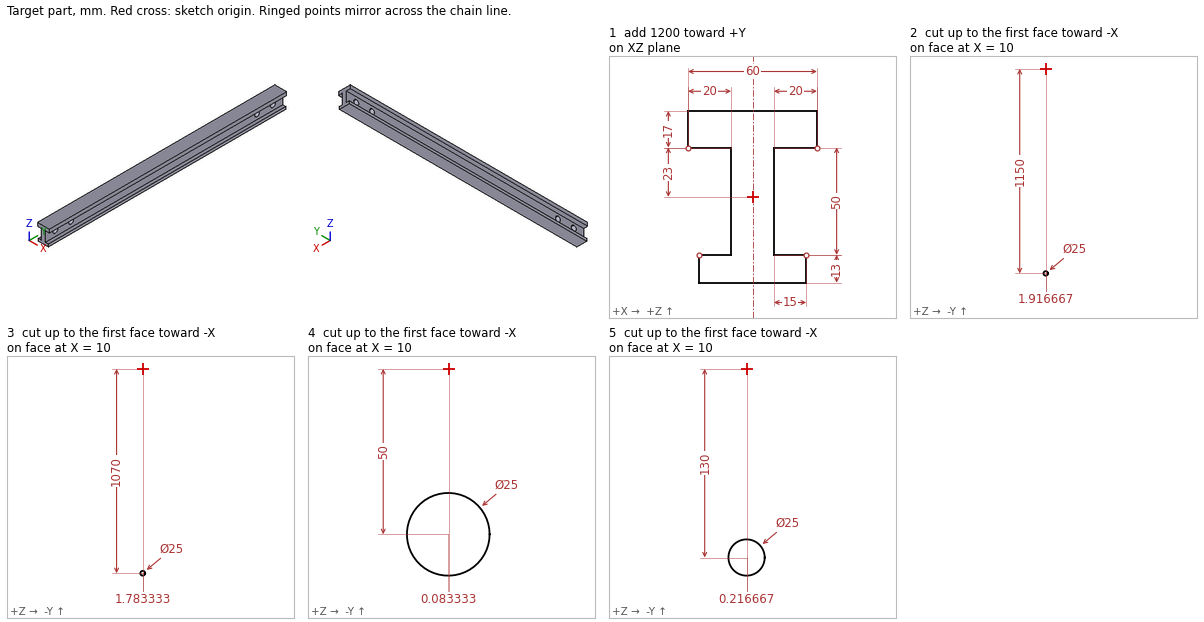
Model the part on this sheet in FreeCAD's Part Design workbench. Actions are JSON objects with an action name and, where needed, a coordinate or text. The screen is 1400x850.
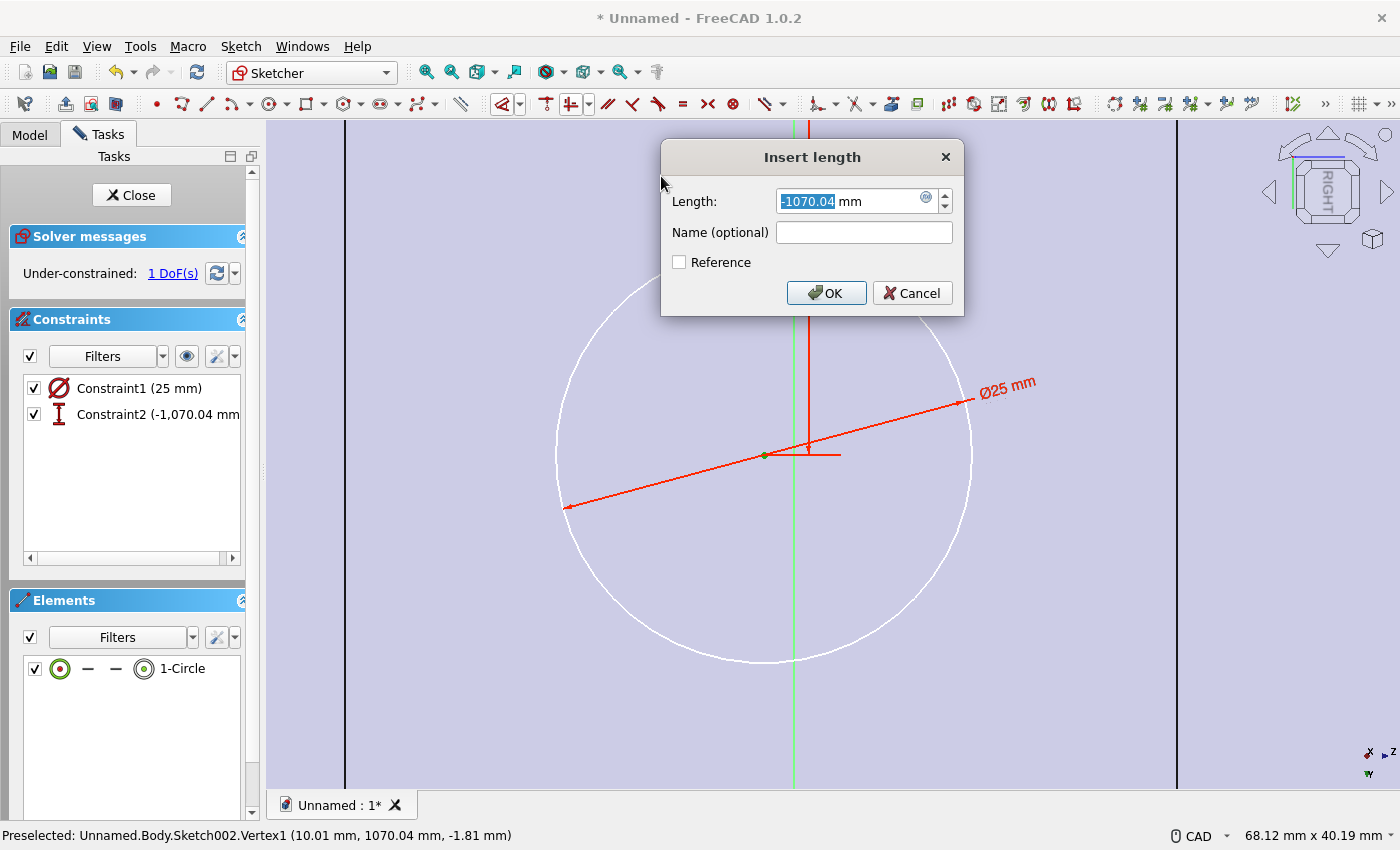
{"action": "type", "text": "-1070"}
{"action": "key", "text": "Return"}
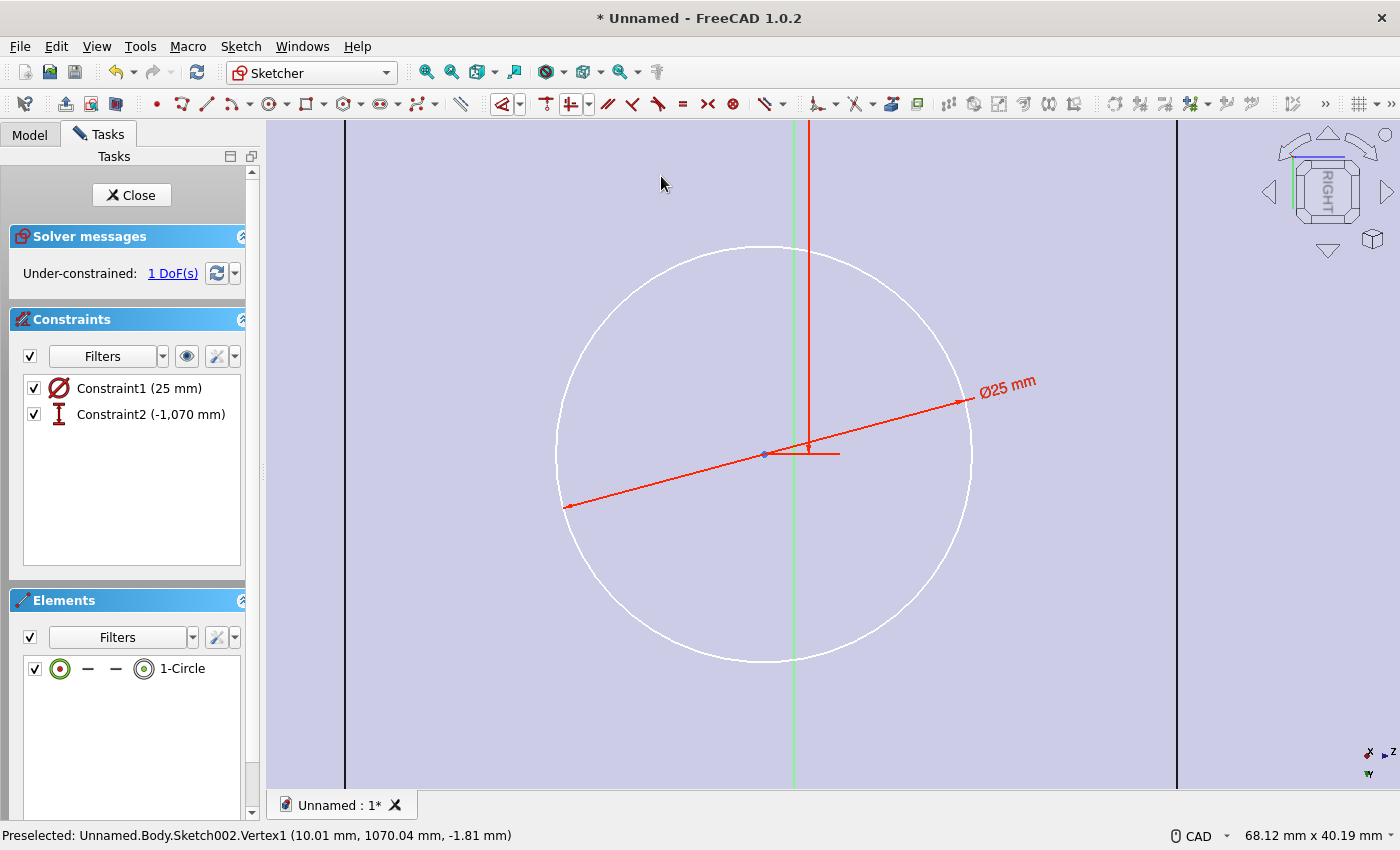
{"action": "scroll", "coordinate": [764, 454], "scroll_direction": "up", "scroll_amount": 2}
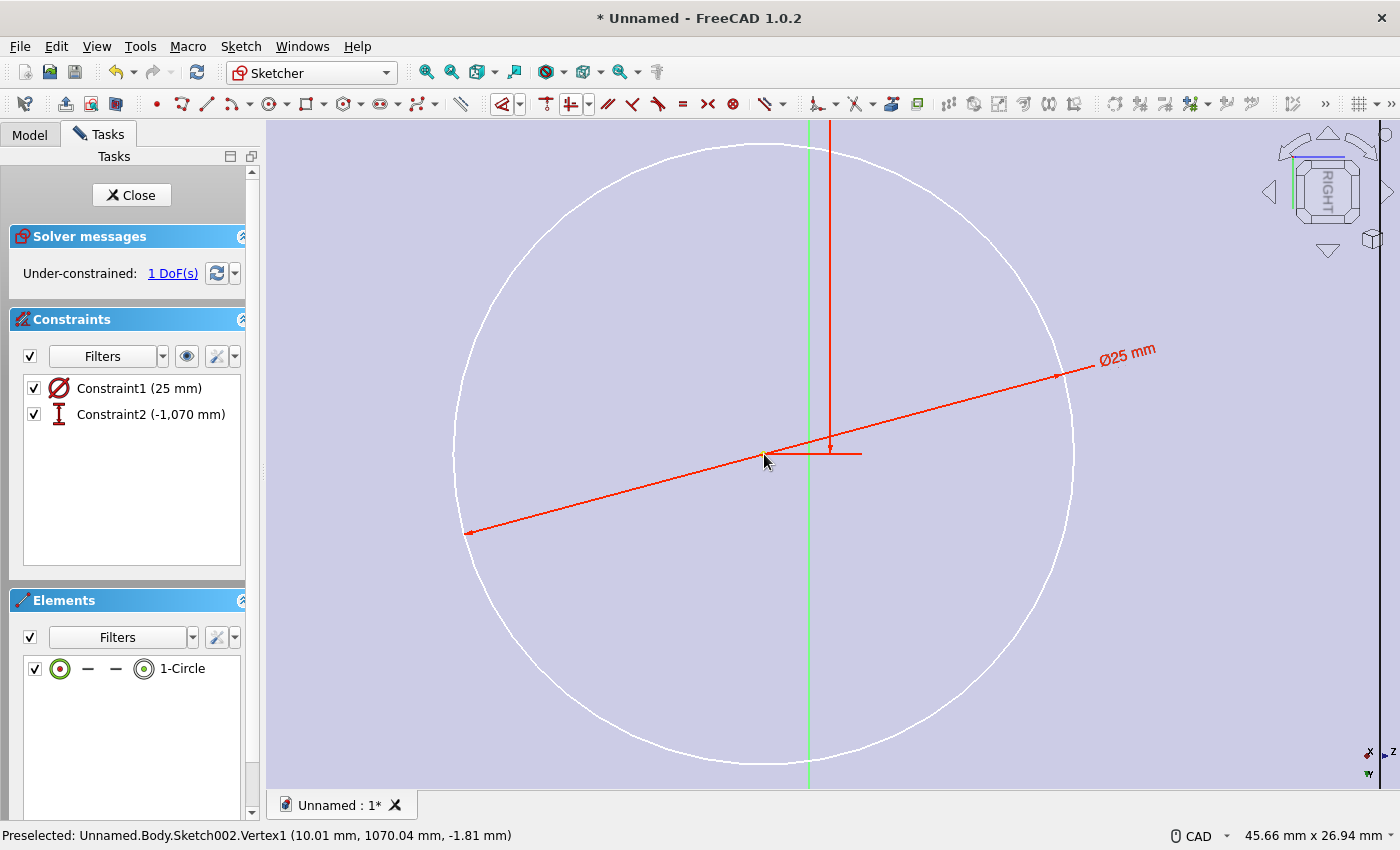
{"action": "left_click", "coordinate": [764, 454]}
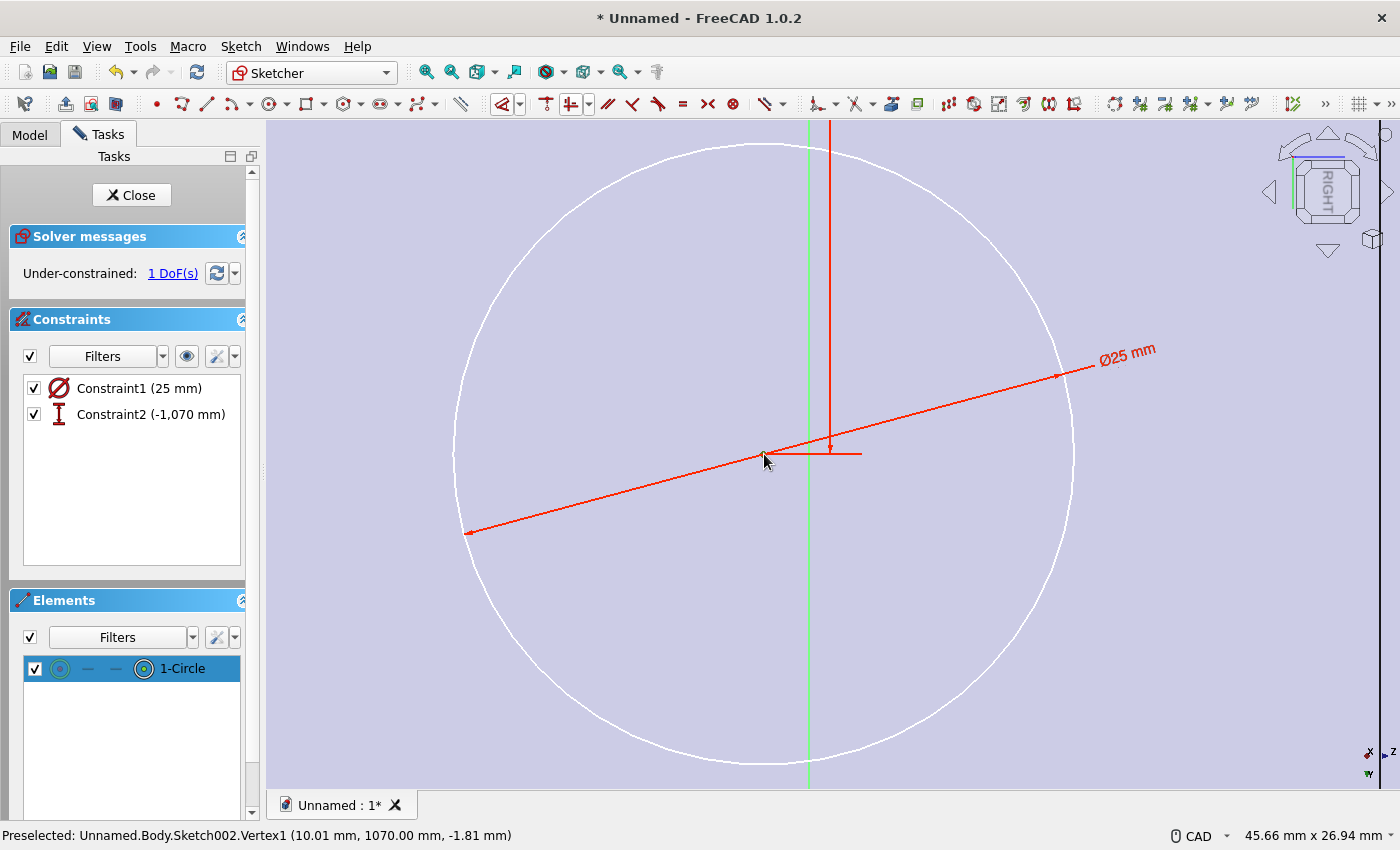
{"action": "key", "text": "l"}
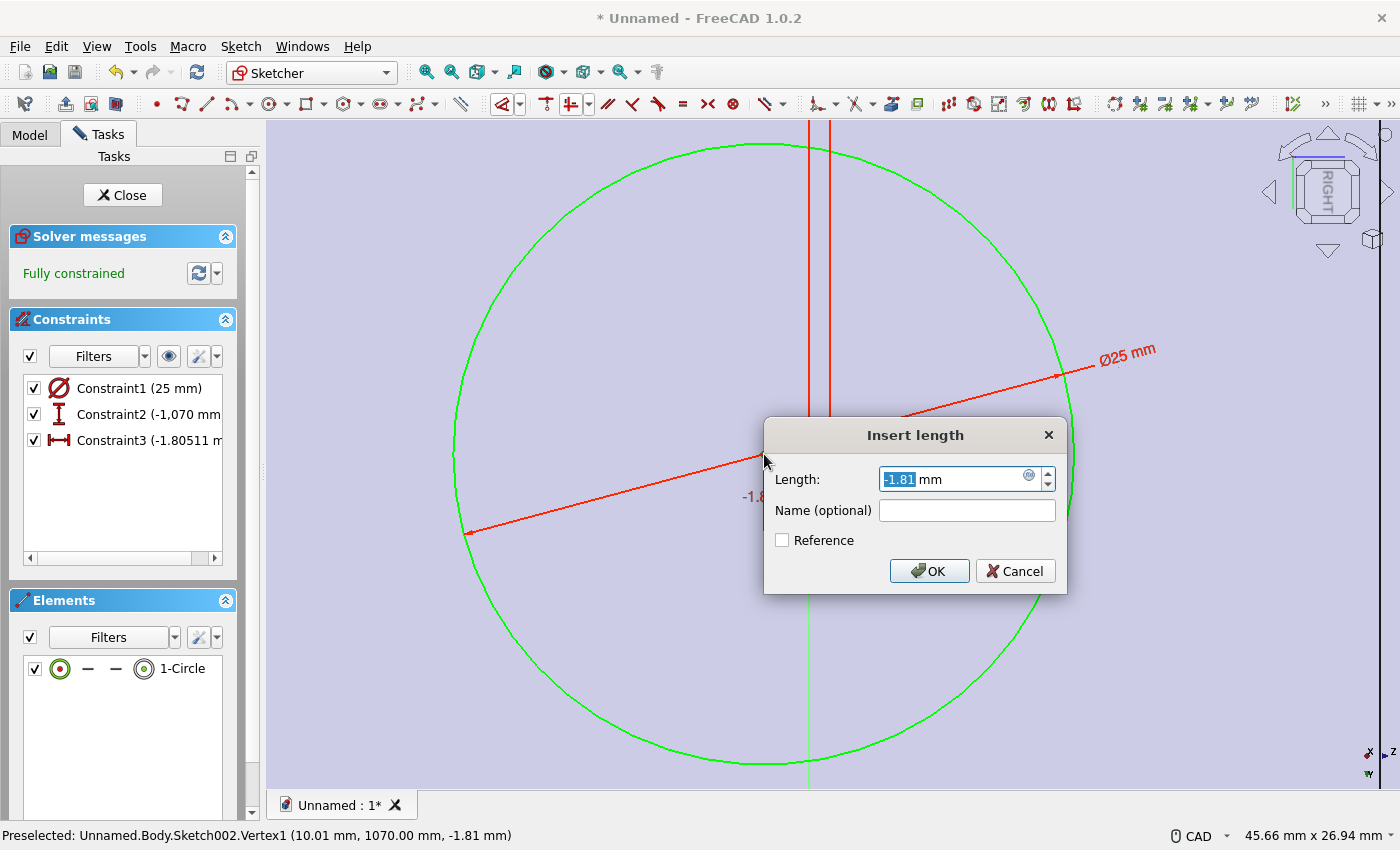
{"action": "type", "text": "-1.783333"}
{"action": "key", "text": "Return"}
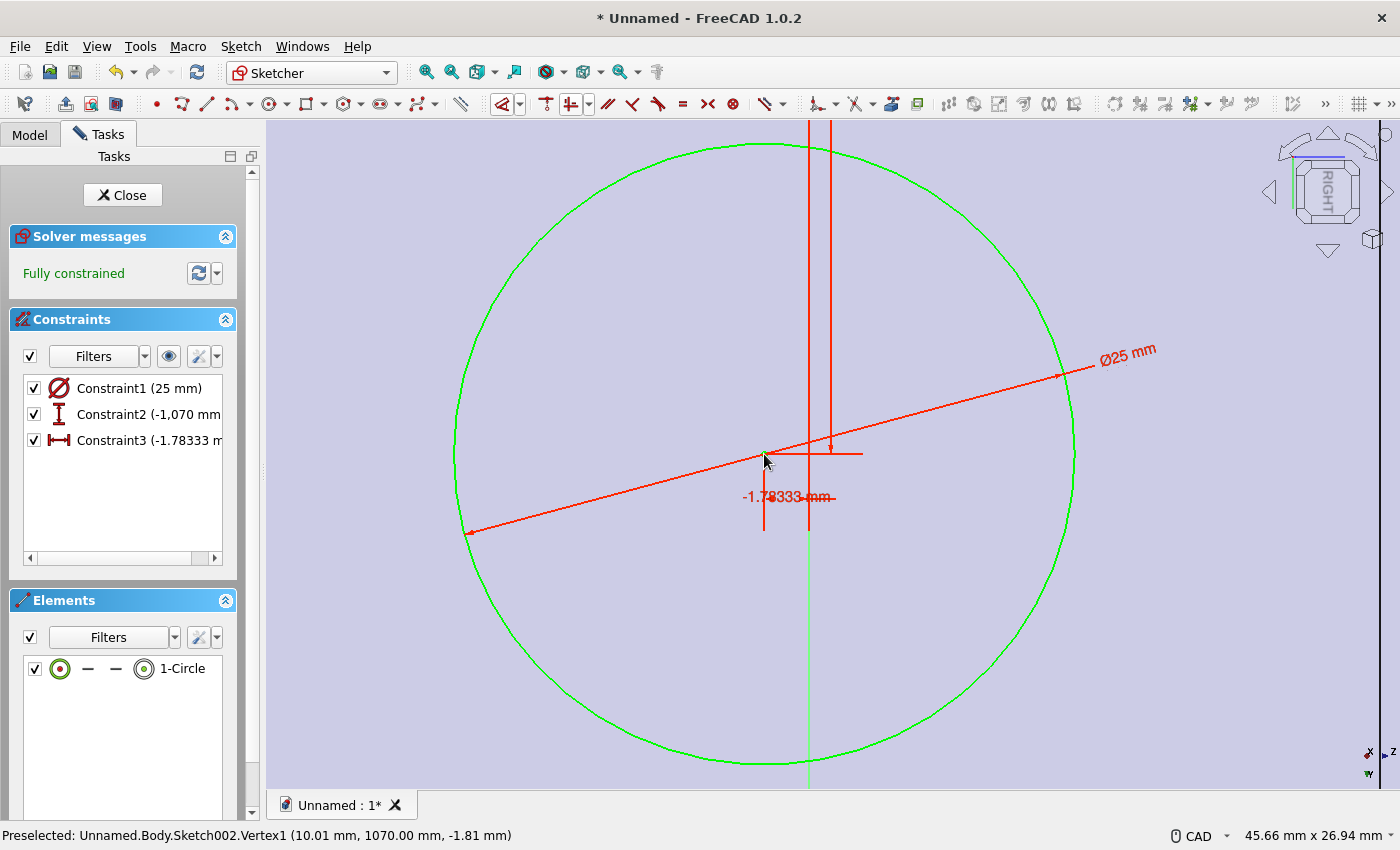
{"action": "left_click", "coordinate": [123, 195]}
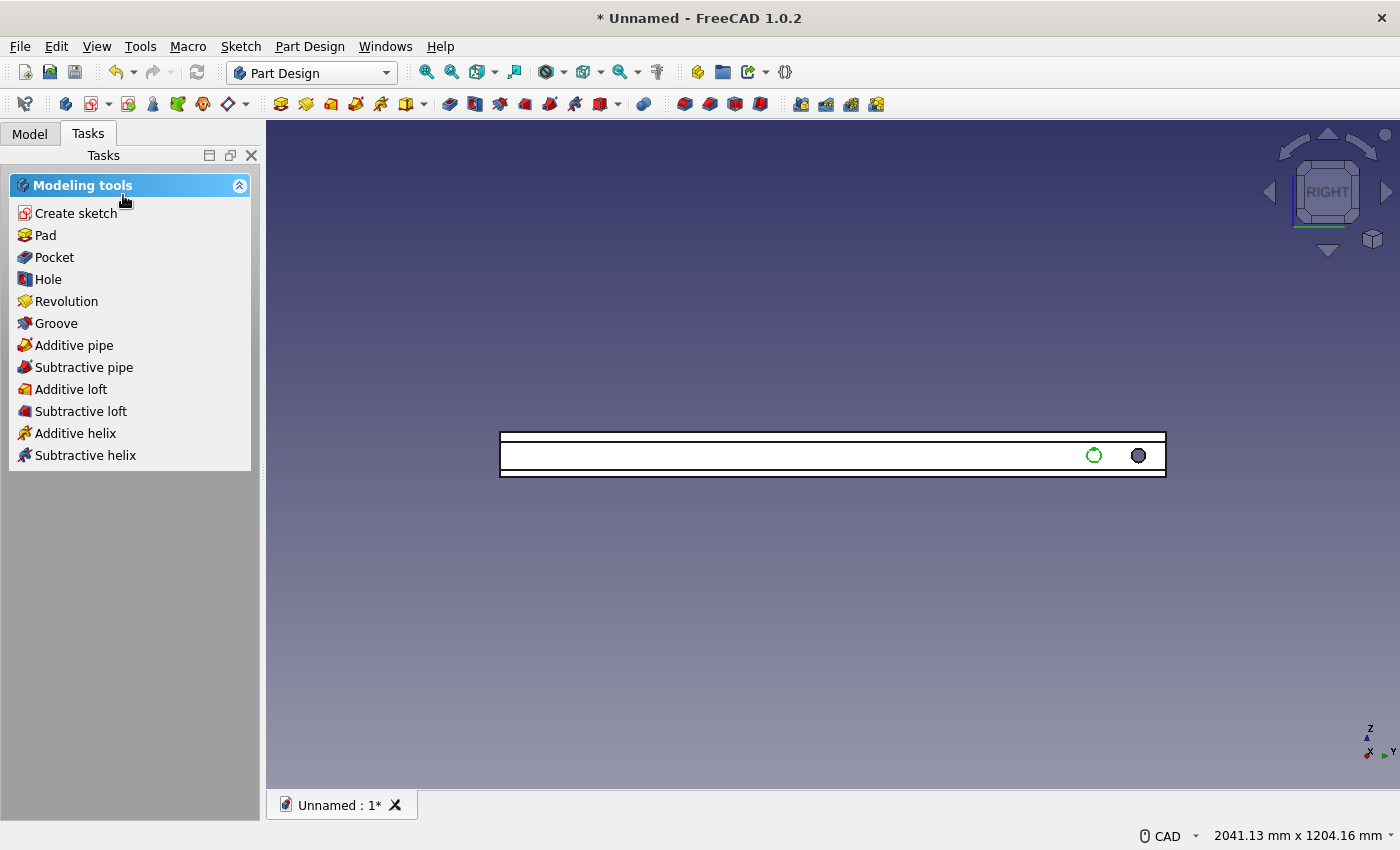
{"action": "left_click", "coordinate": [450, 104]}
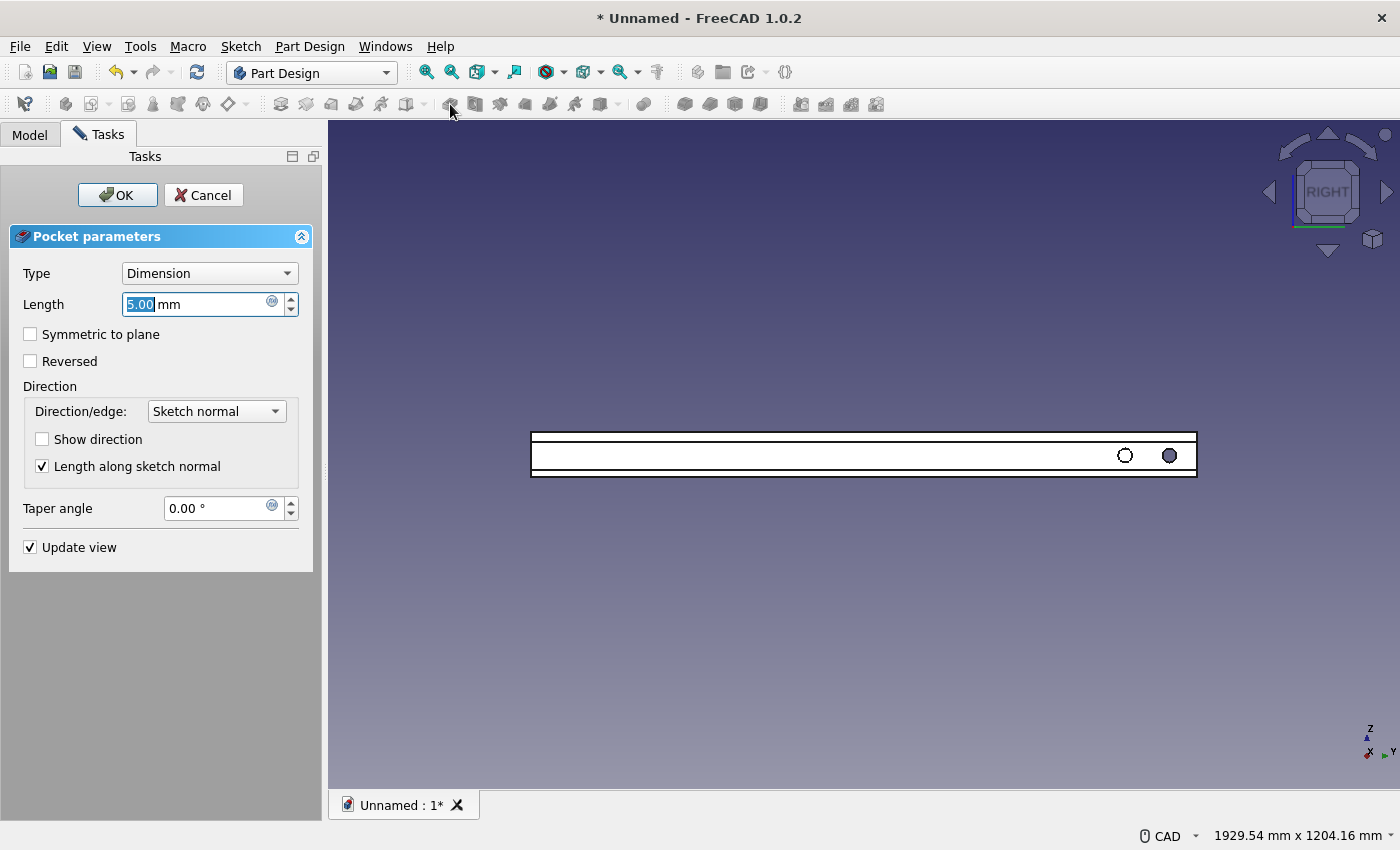
{"action": "left_click", "coordinate": [210, 274]}